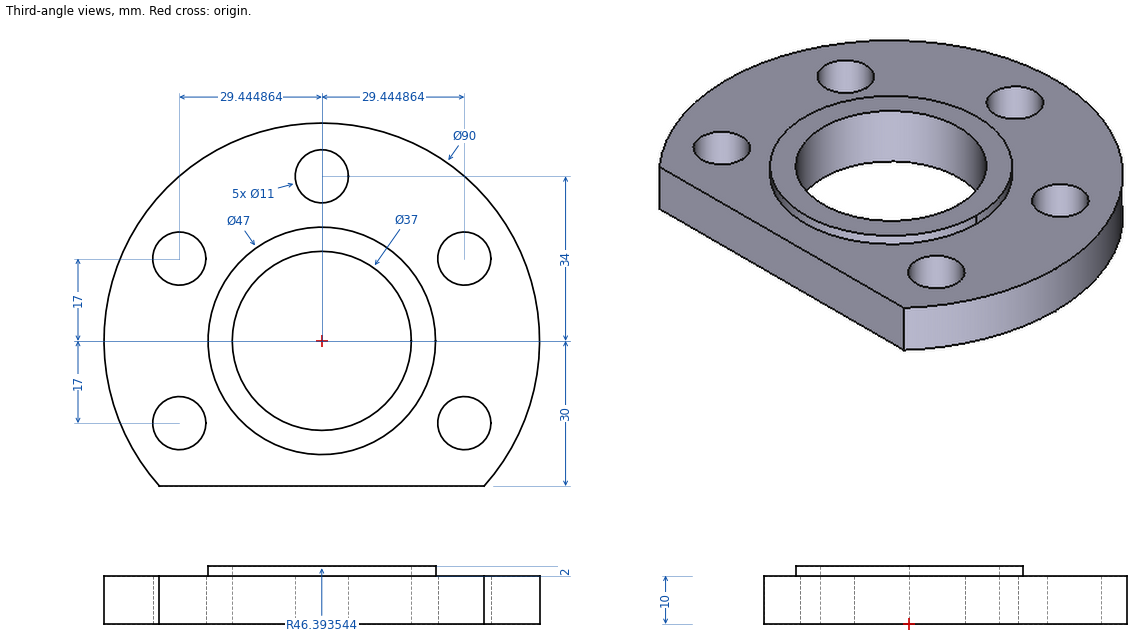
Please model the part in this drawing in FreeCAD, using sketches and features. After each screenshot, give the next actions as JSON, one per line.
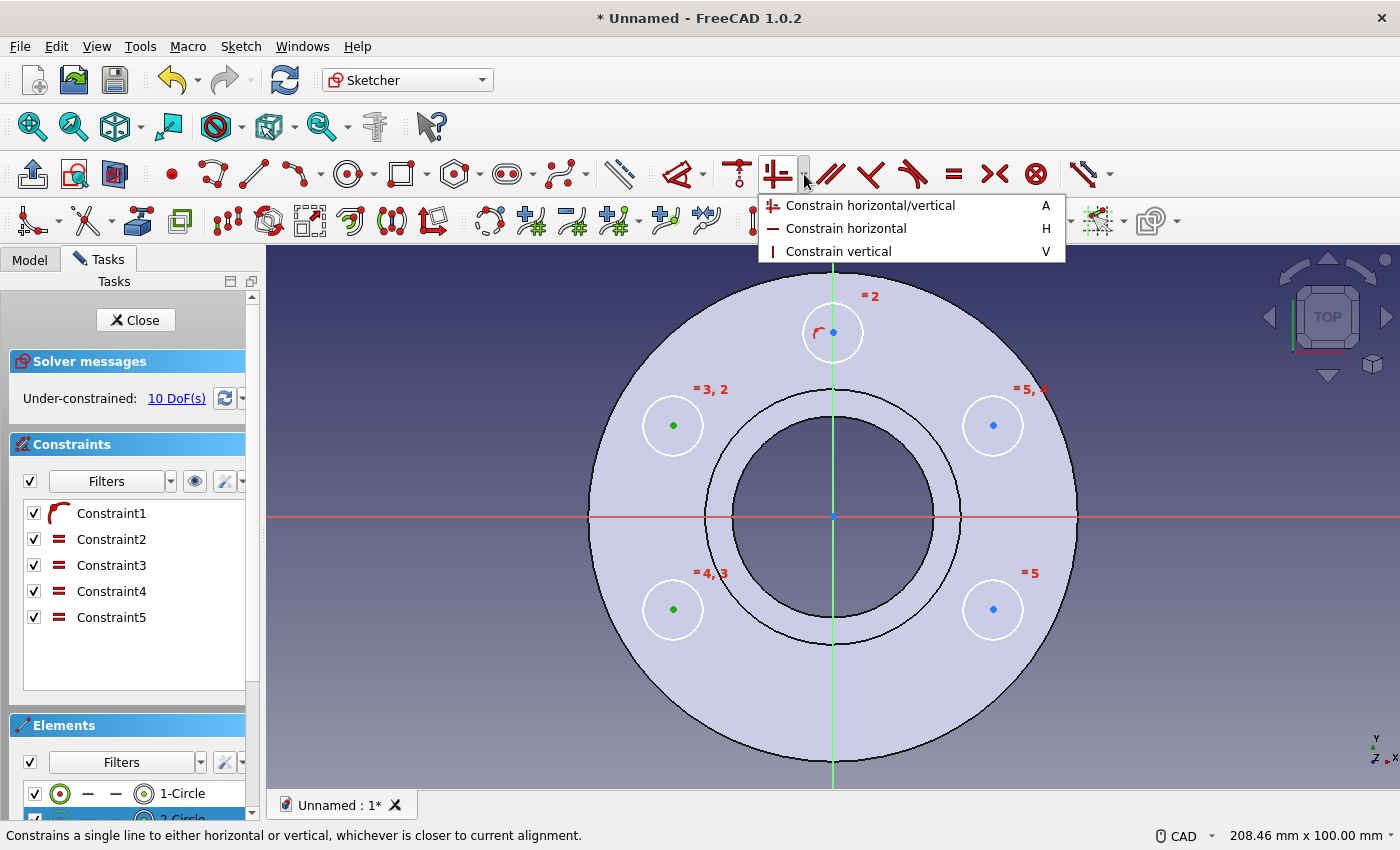
{"action": "left_click", "coordinate": [912, 252]}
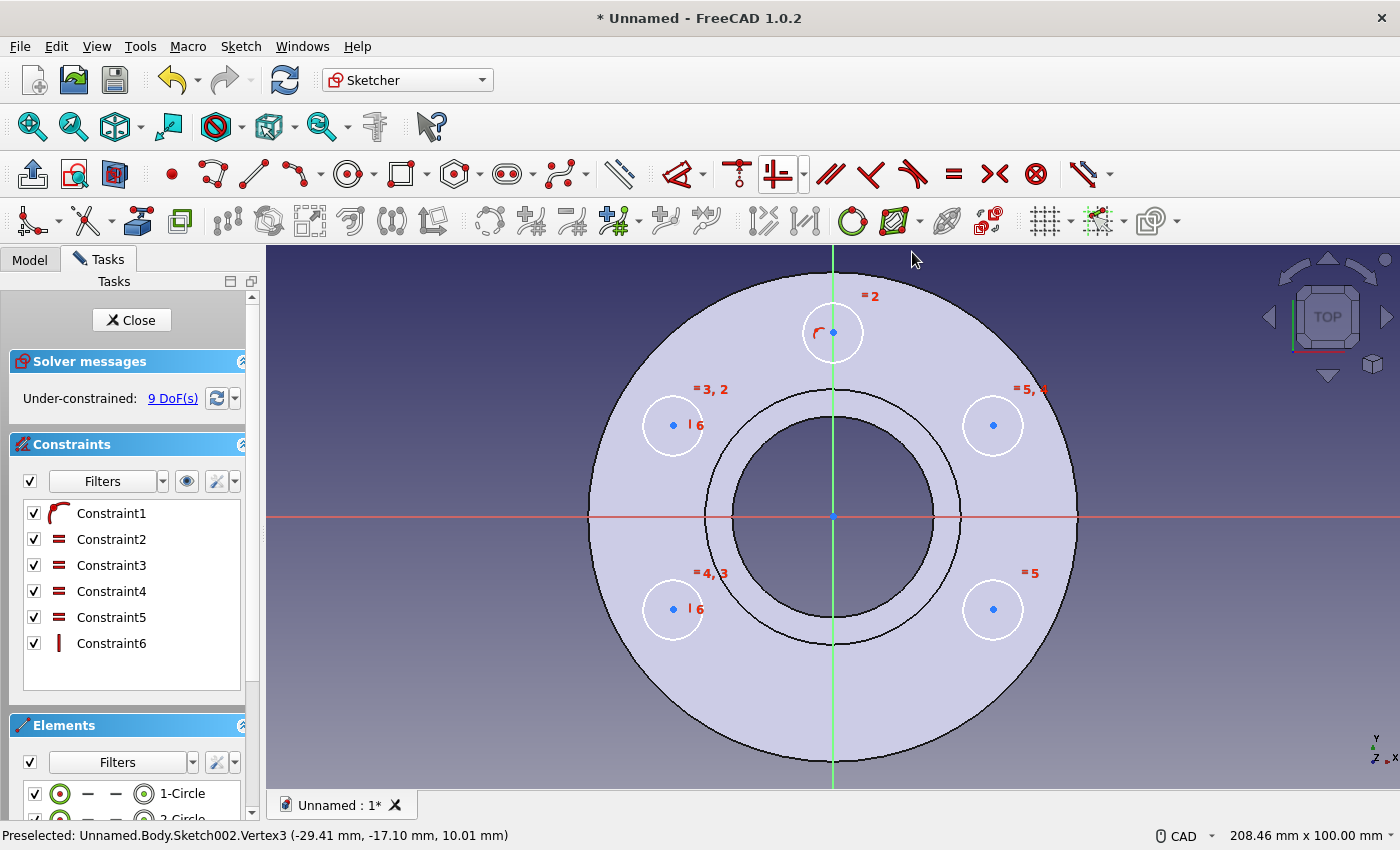
{"action": "left_click", "coordinate": [673, 426]}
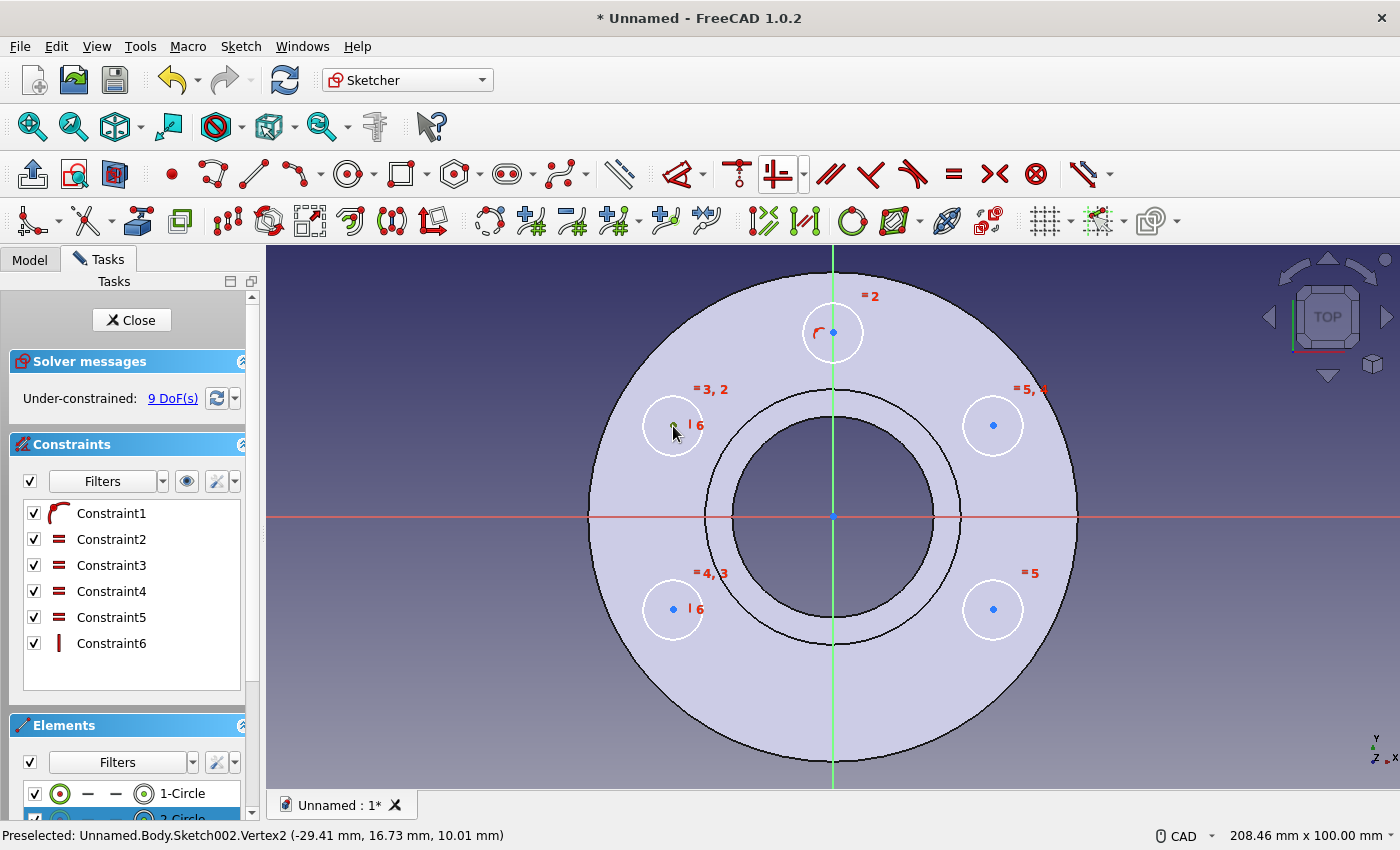
{"action": "left_click", "coordinate": [993, 426]}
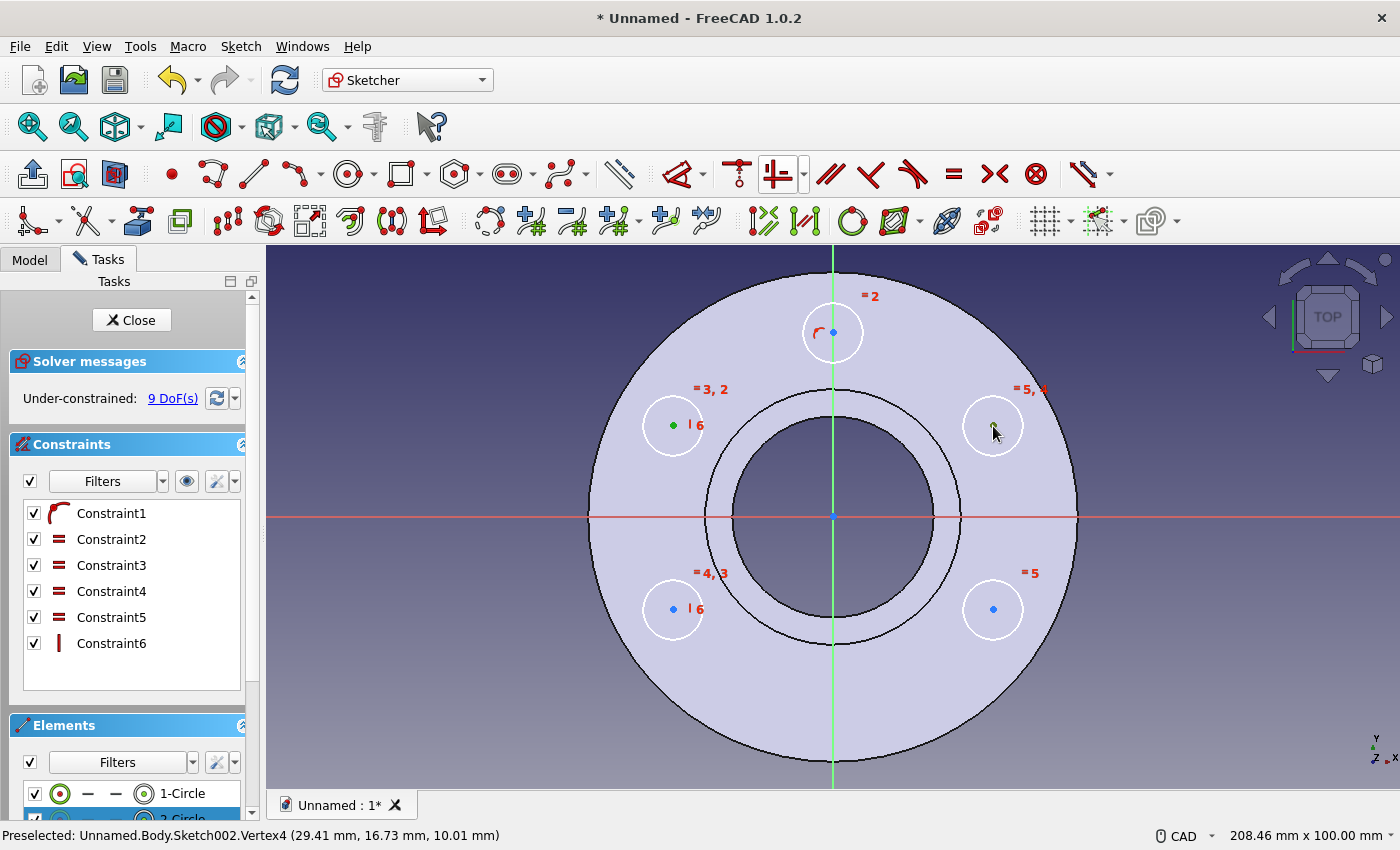
{"action": "key", "text": "h"}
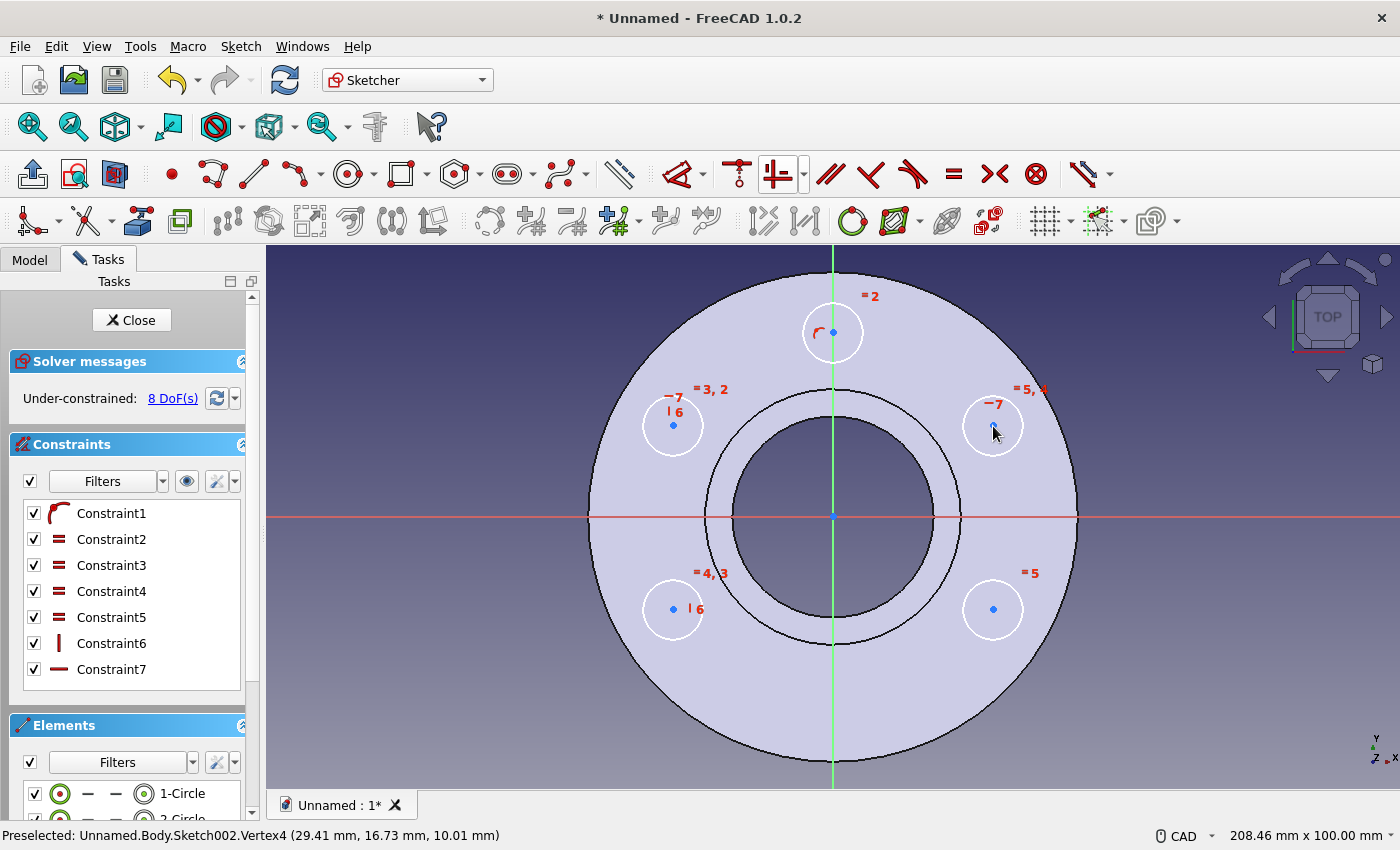
{"action": "left_click", "coordinate": [993, 426]}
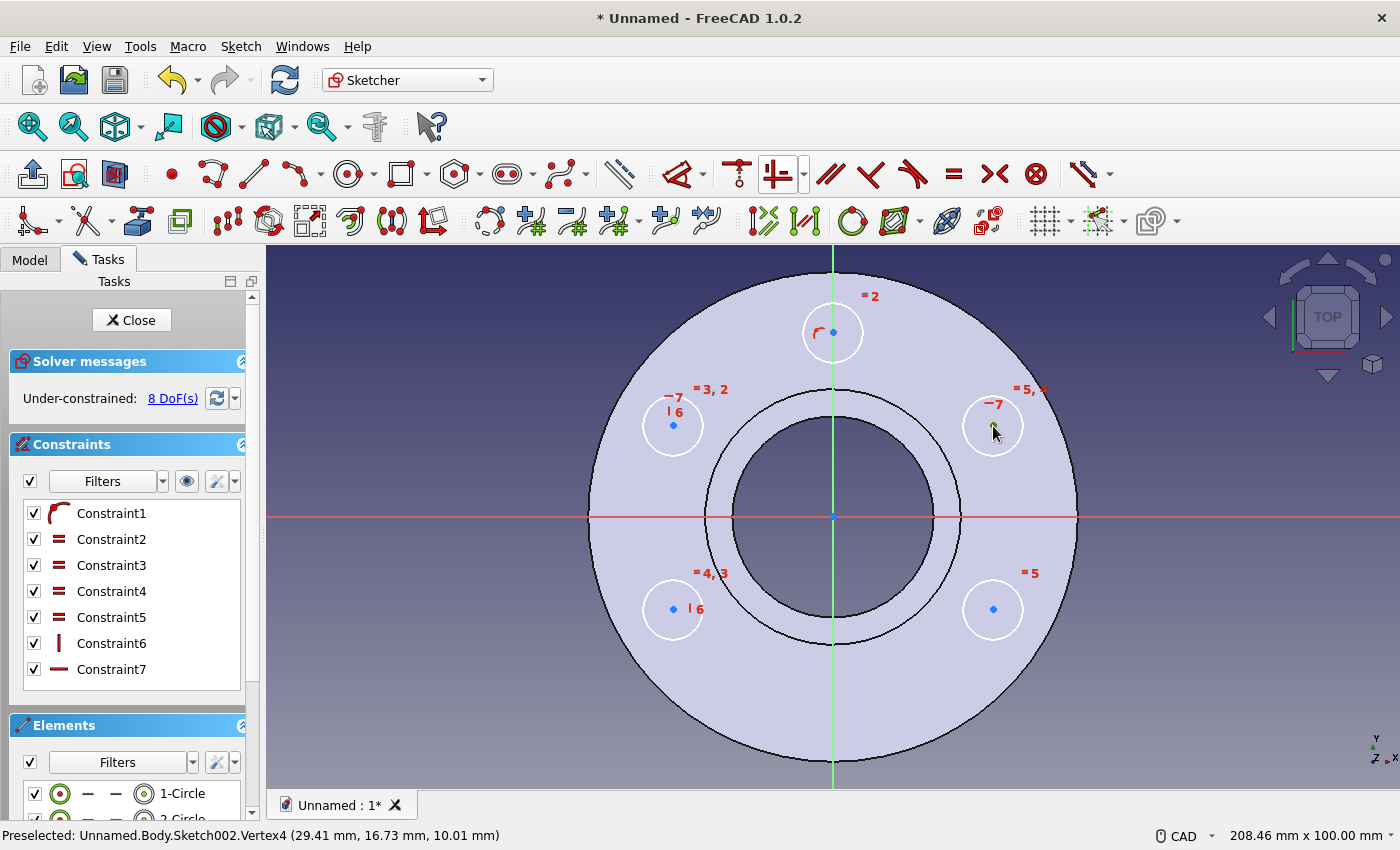
{"action": "left_click", "coordinate": [993, 610]}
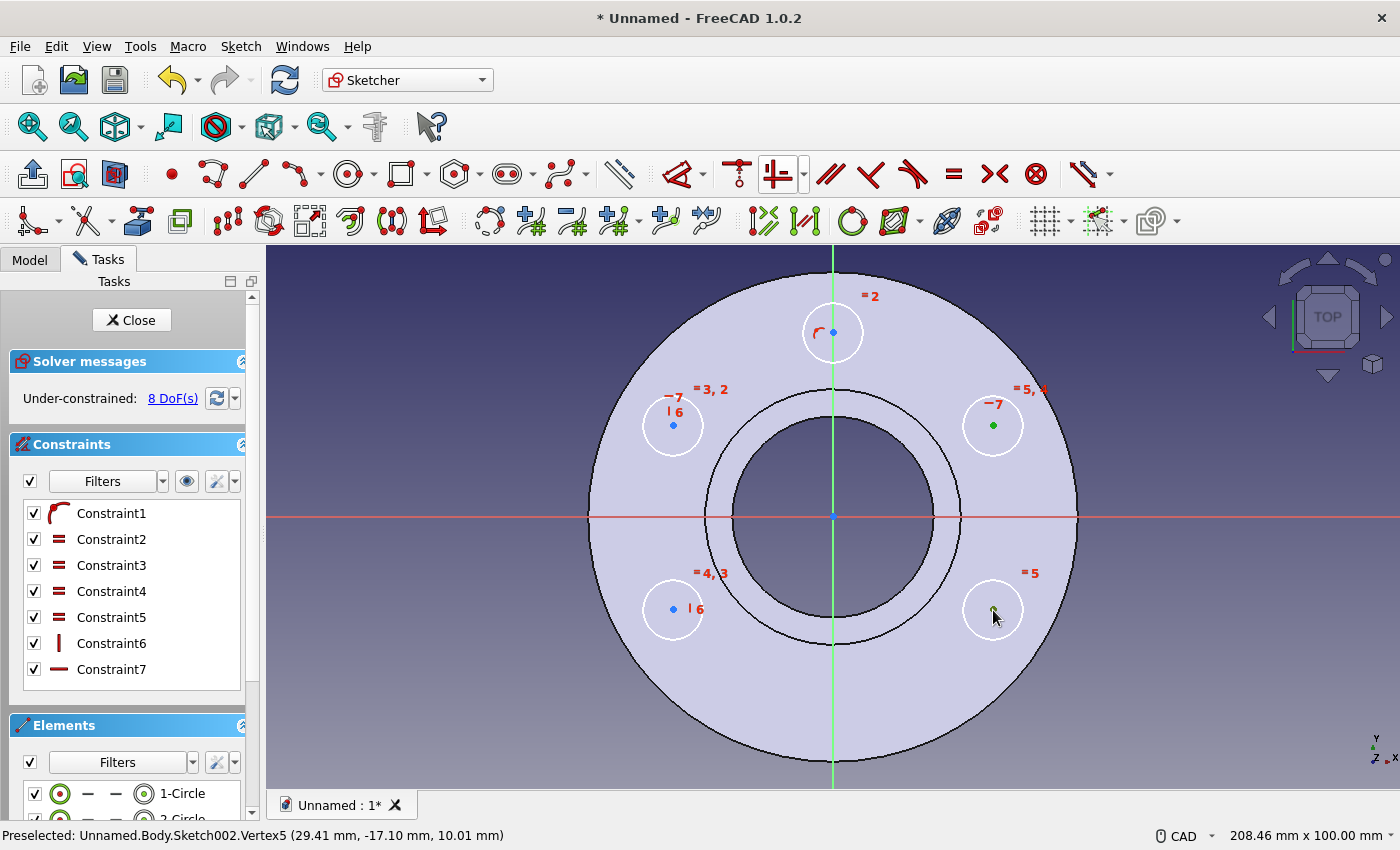
{"action": "left_click", "coordinate": [804, 174]}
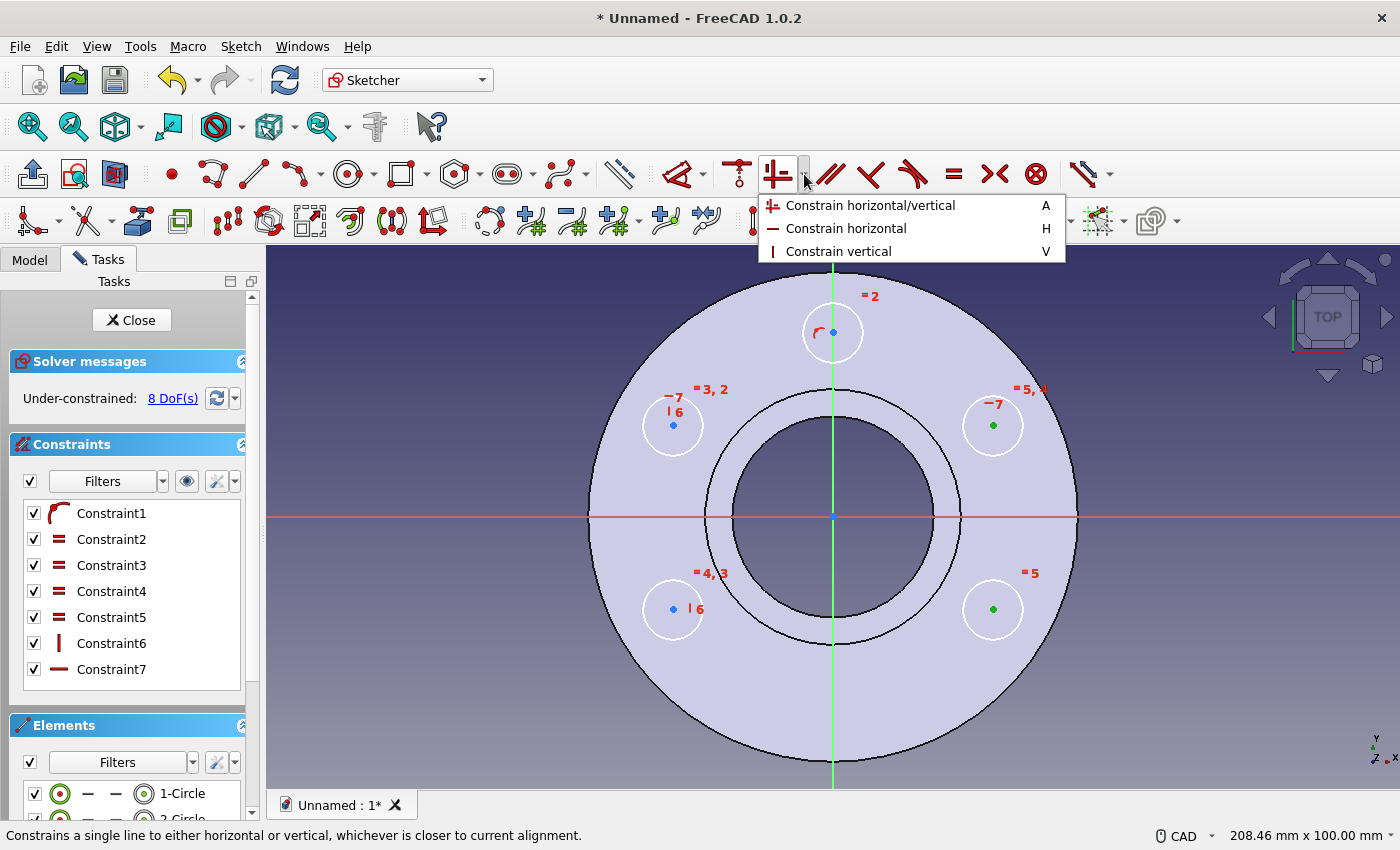
{"action": "left_click", "coordinate": [912, 252]}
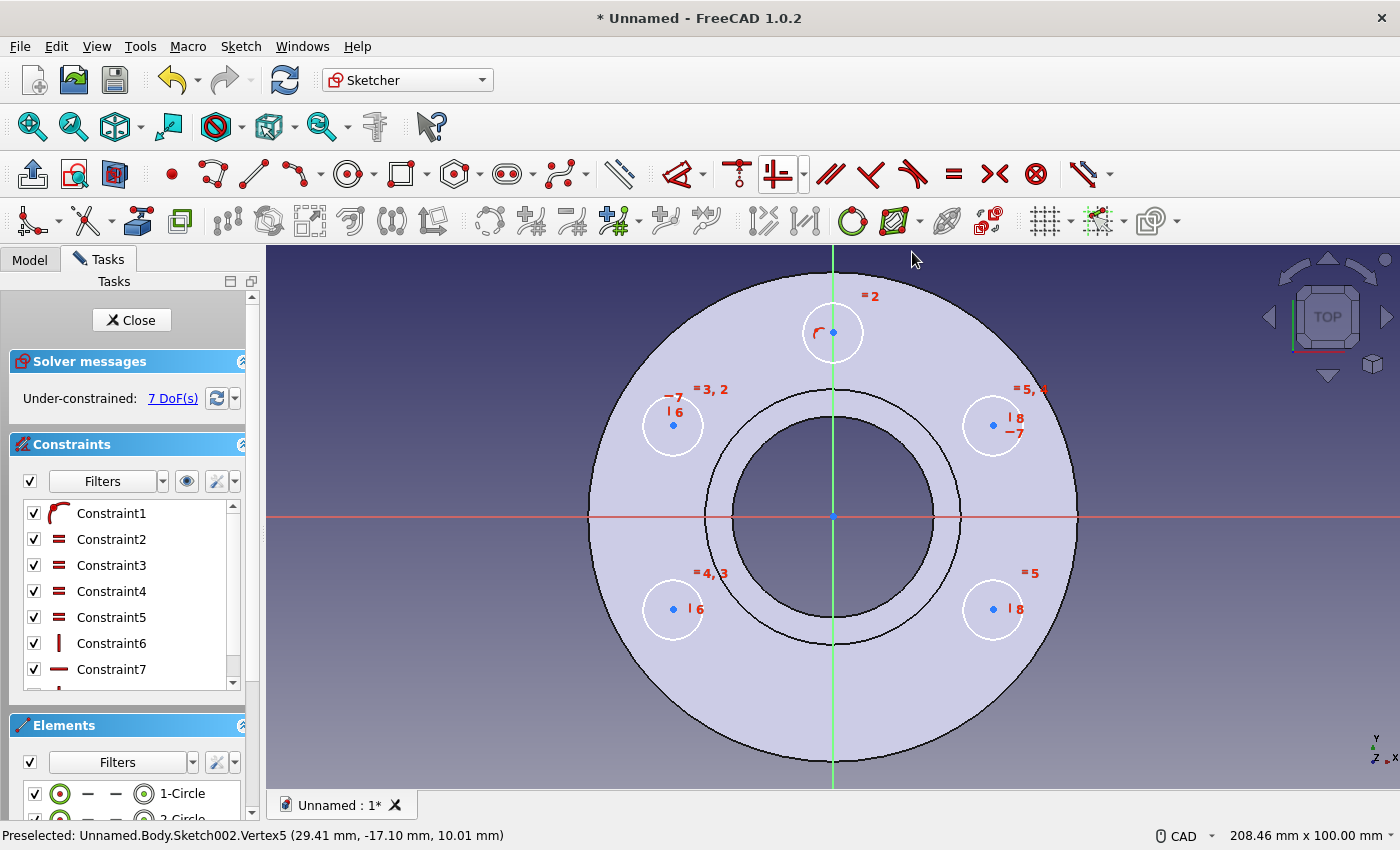
{"action": "left_click", "coordinate": [673, 610]}